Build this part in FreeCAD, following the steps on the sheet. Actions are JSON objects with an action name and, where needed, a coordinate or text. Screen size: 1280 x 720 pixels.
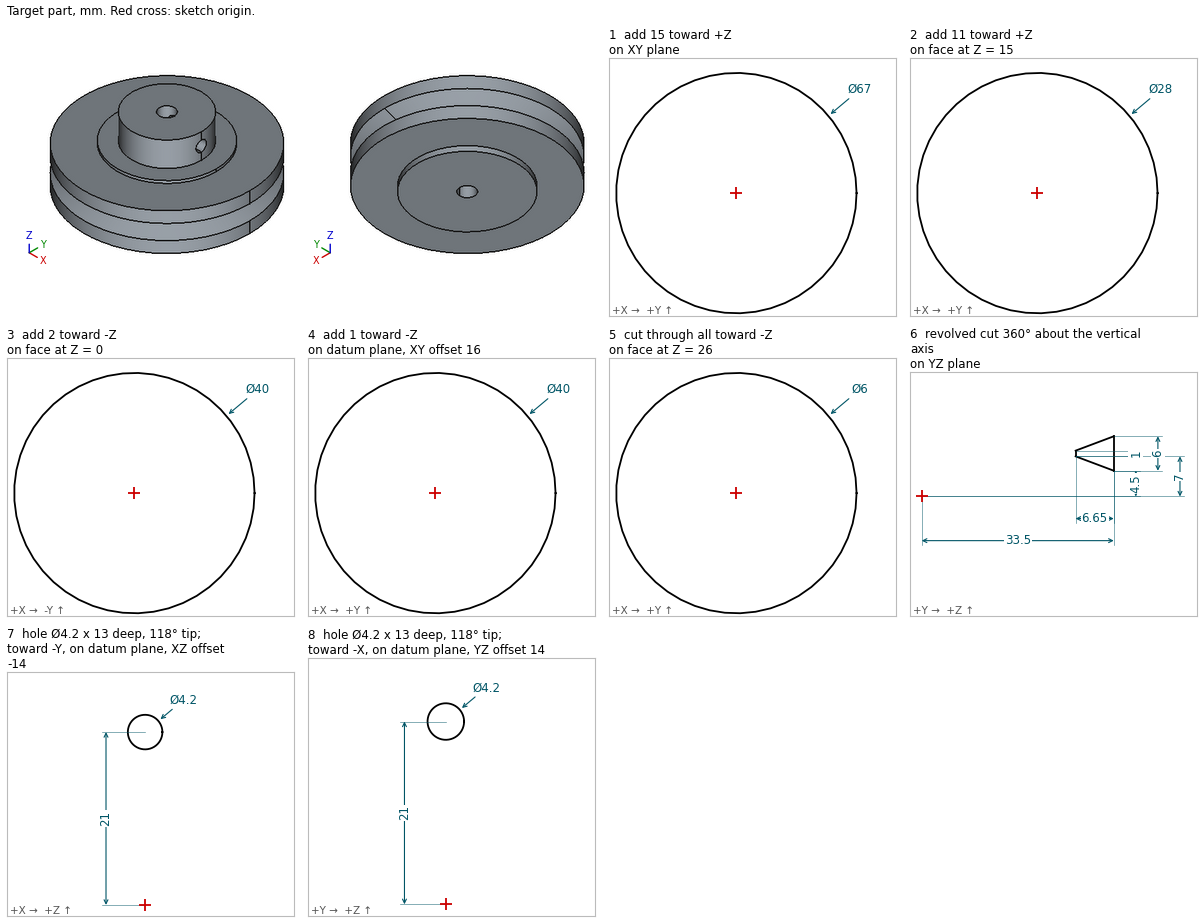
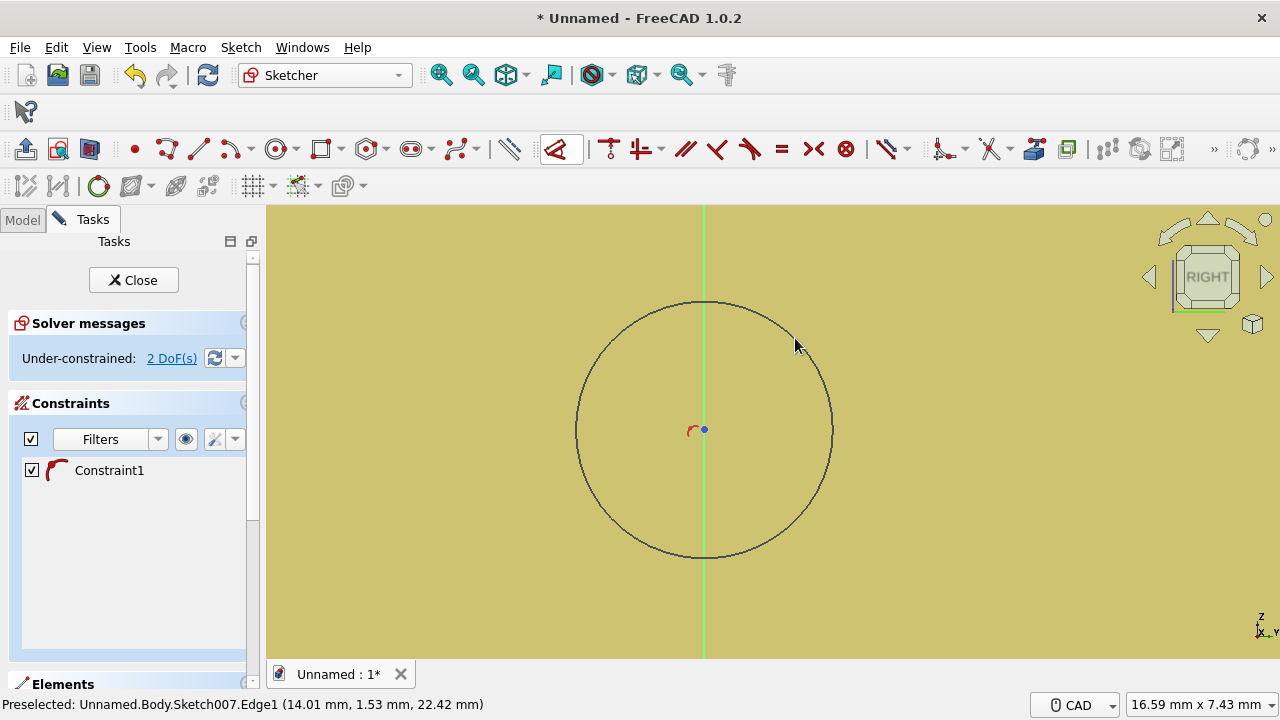
{"action": "left_click", "coordinate": [795, 339]}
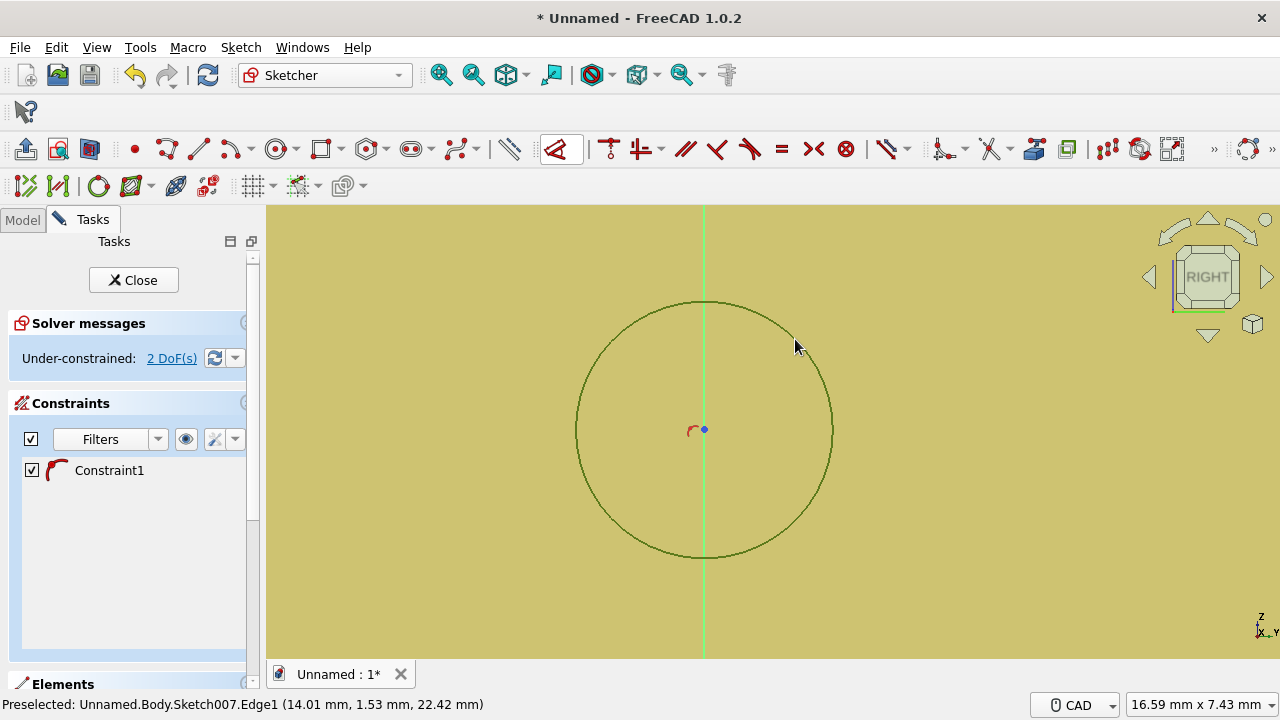
{"action": "key", "text": "k o"}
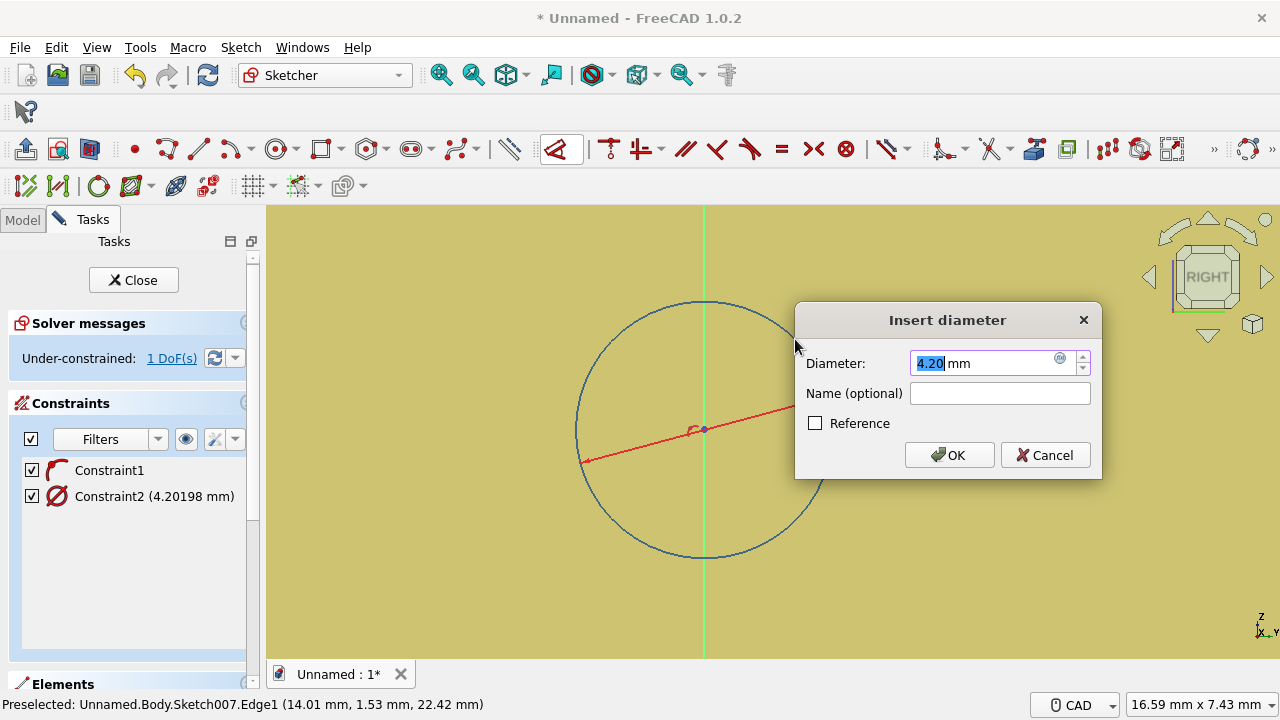
{"action": "type", "text": "4.2"}
{"action": "key", "text": "Return"}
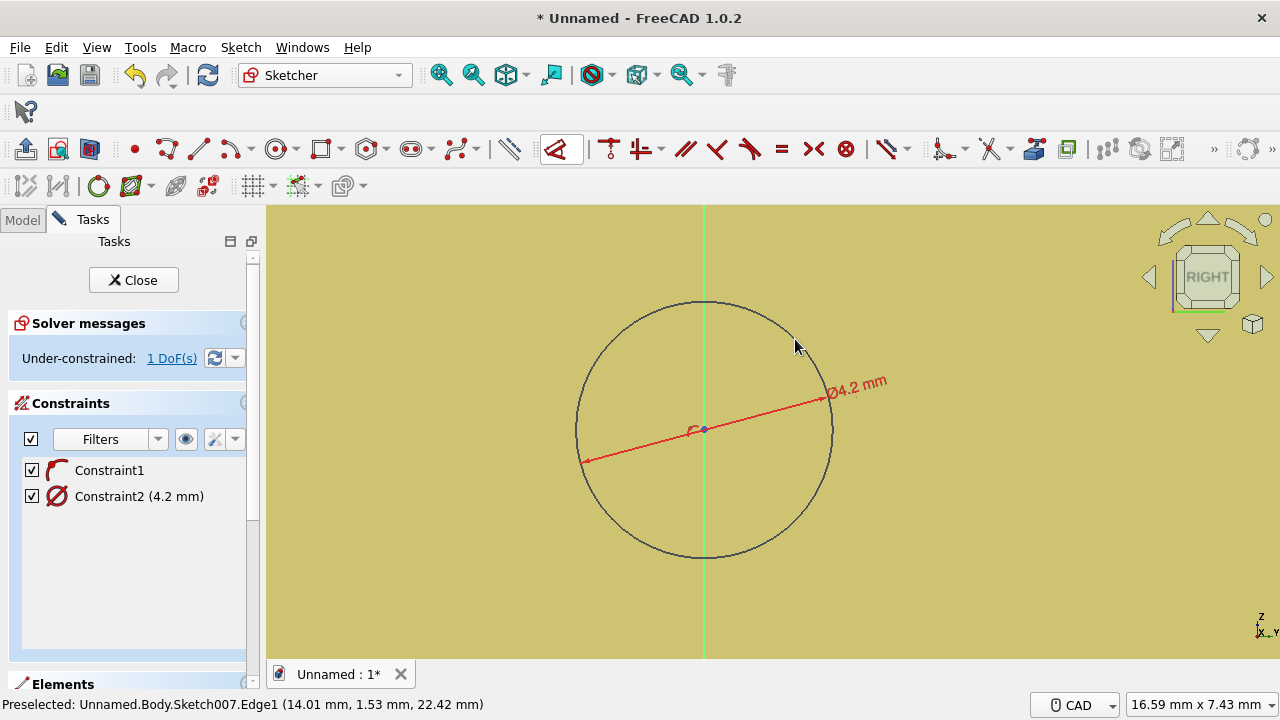
{"action": "left_click", "coordinate": [704, 430]}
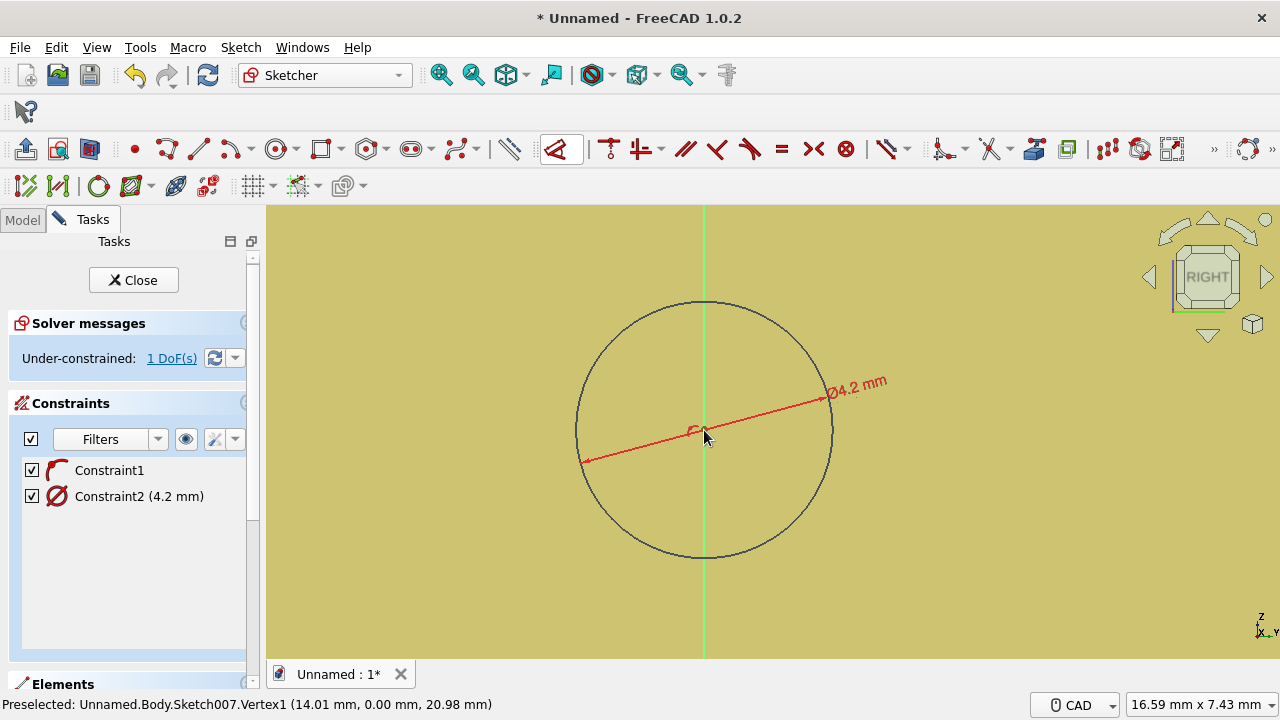
{"action": "key", "text": "i"}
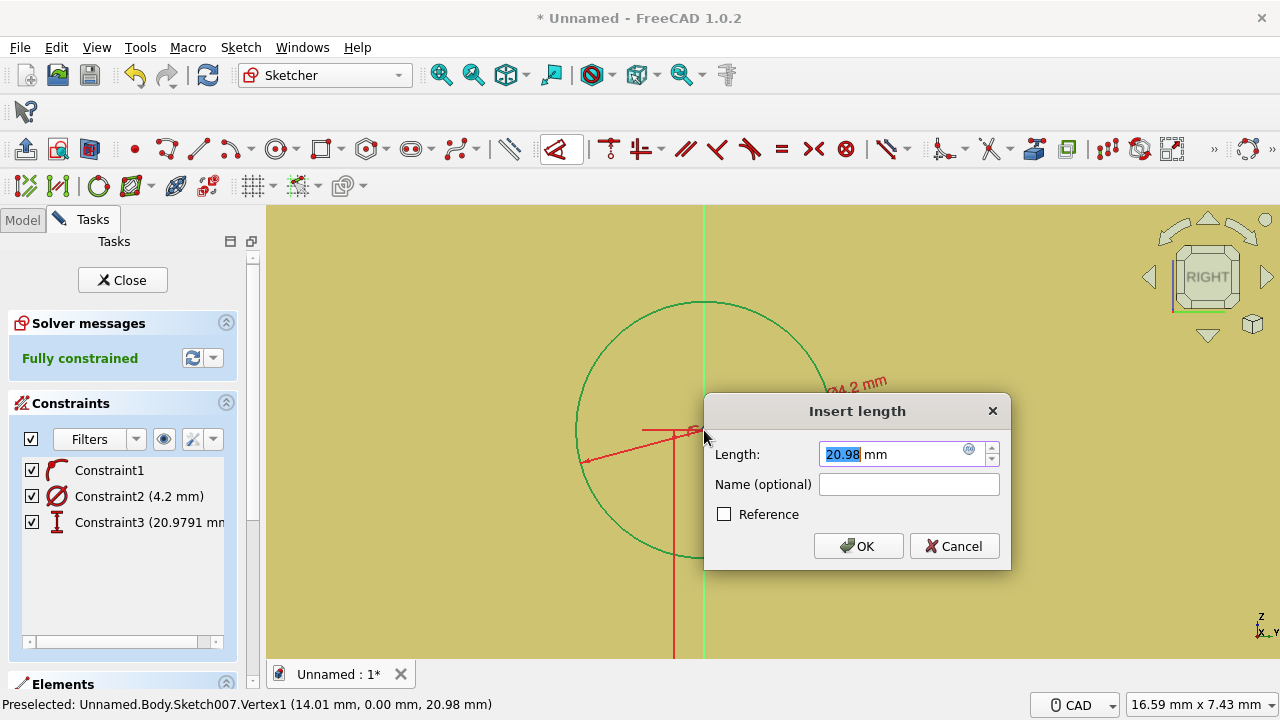
{"action": "type", "text": "21"}
{"action": "key", "text": "Return"}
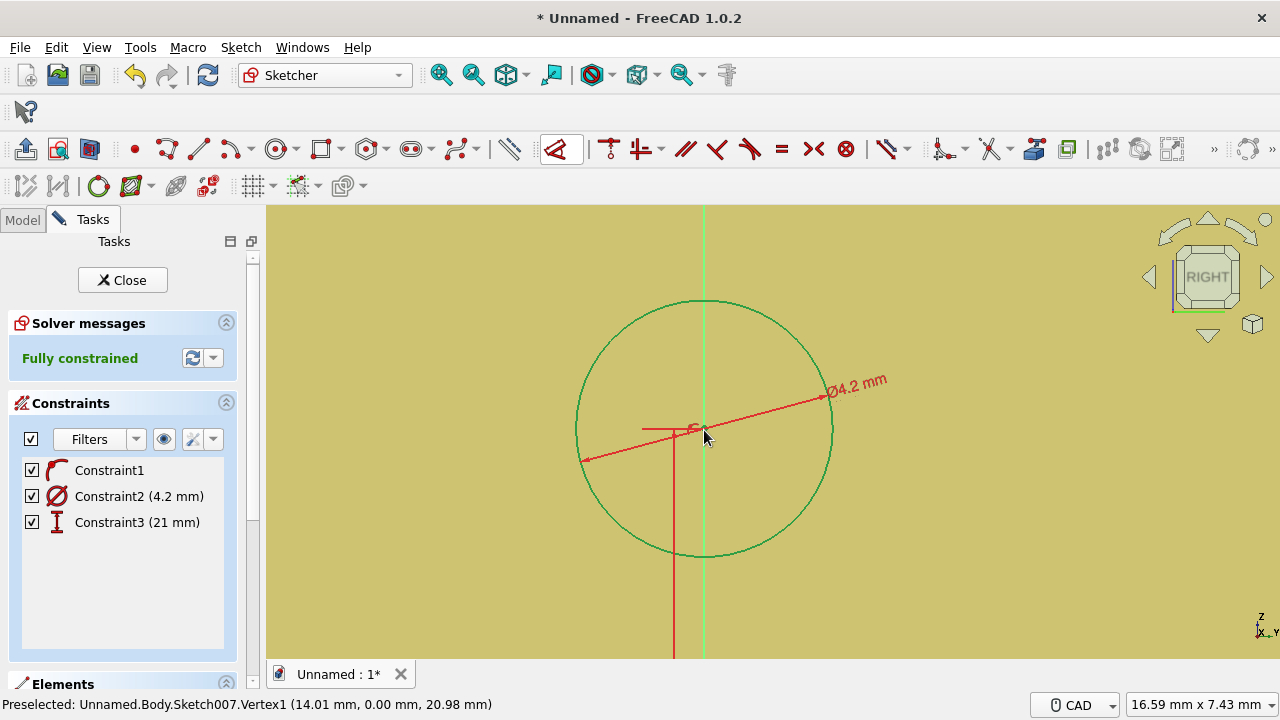
{"action": "left_click", "coordinate": [123, 280]}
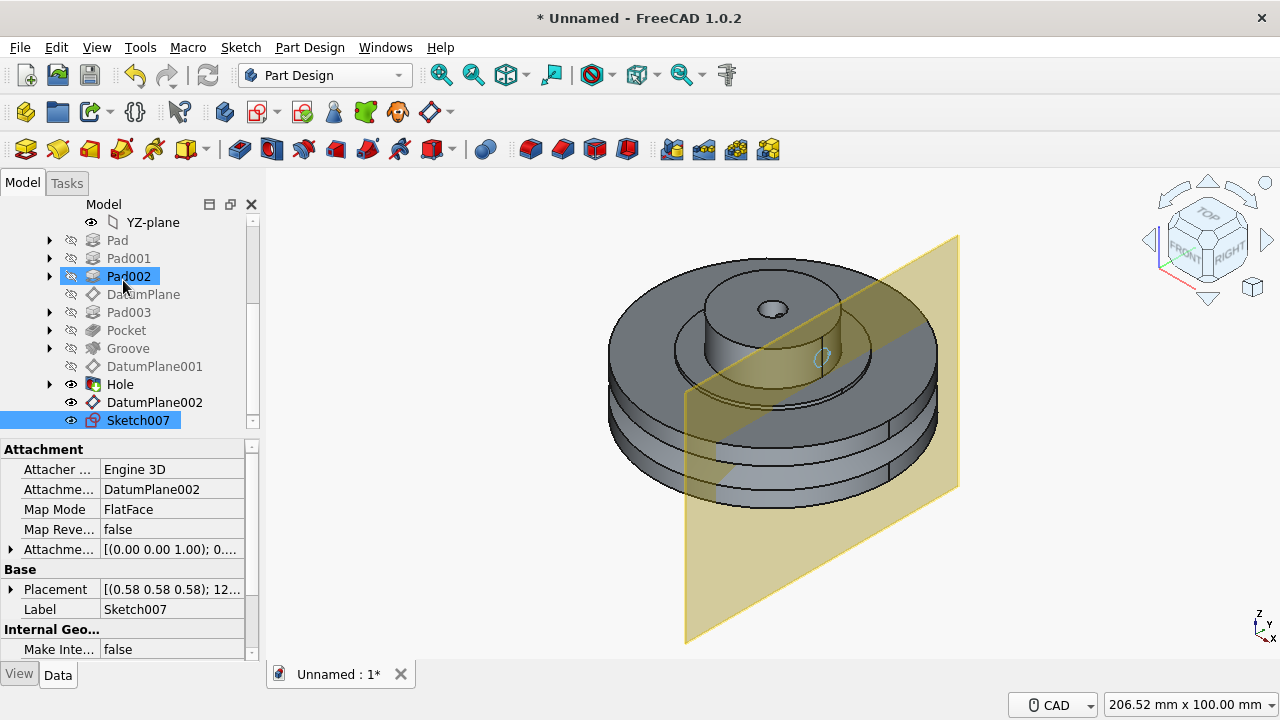
{"action": "left_click", "coordinate": [272, 150]}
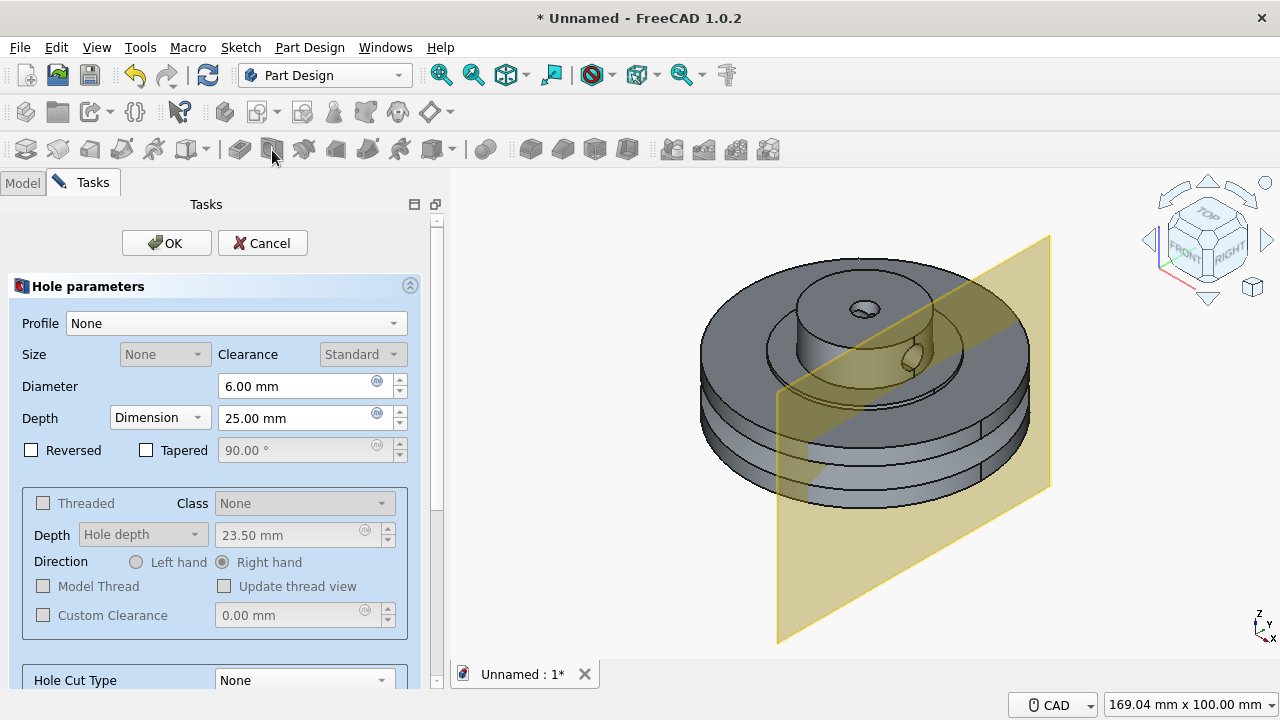
{"action": "triple_click", "coordinate": [305, 386]}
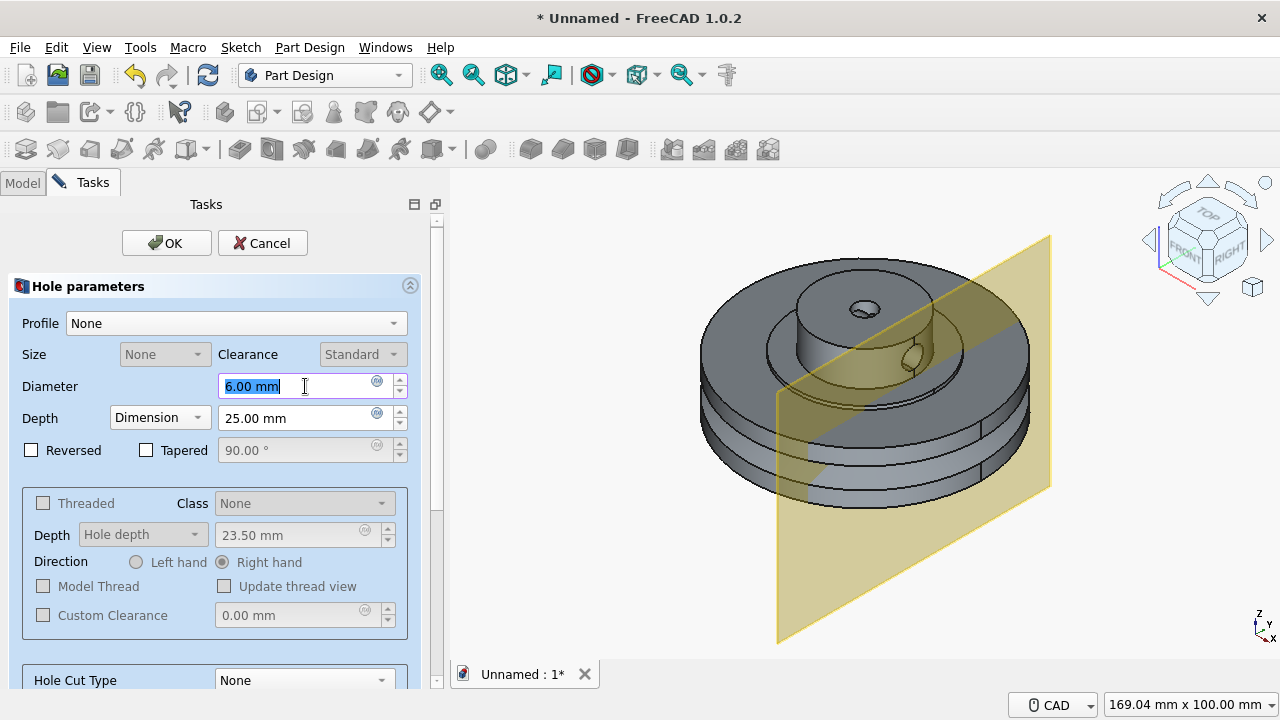
{"action": "type", "text": "4.2"}
{"action": "key", "text": "Tab"}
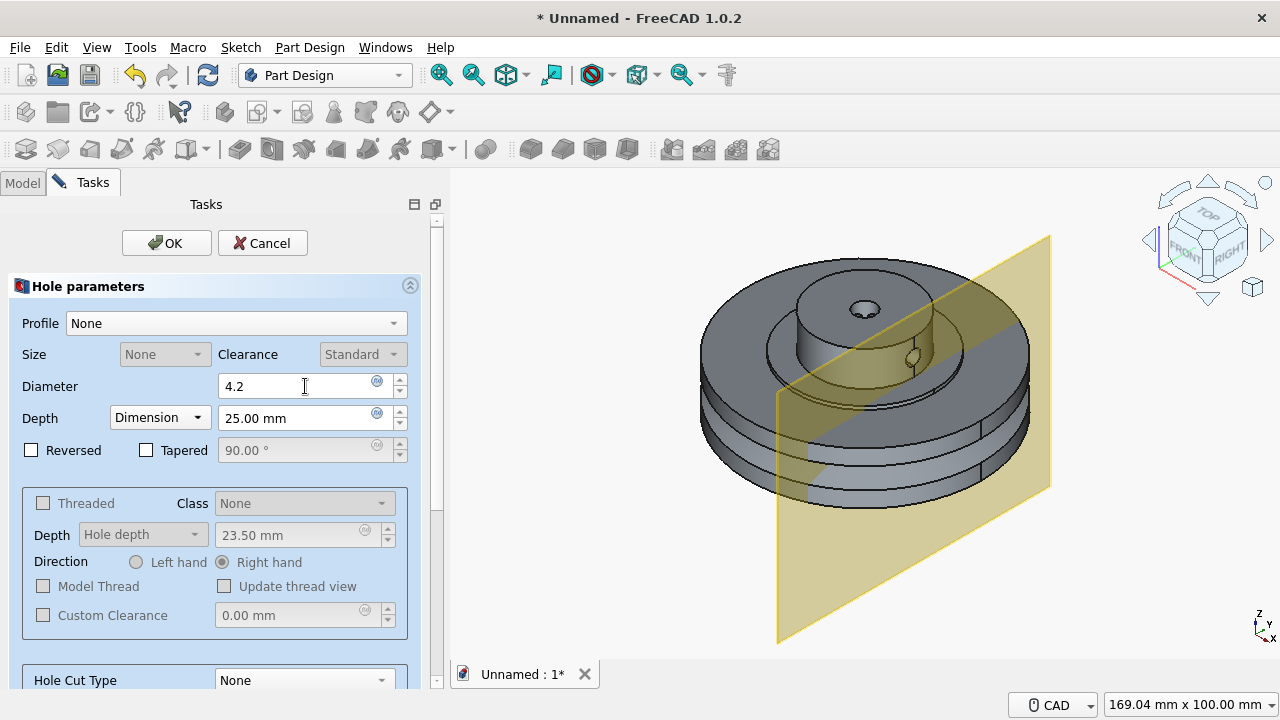
{"action": "triple_click", "coordinate": [305, 418]}